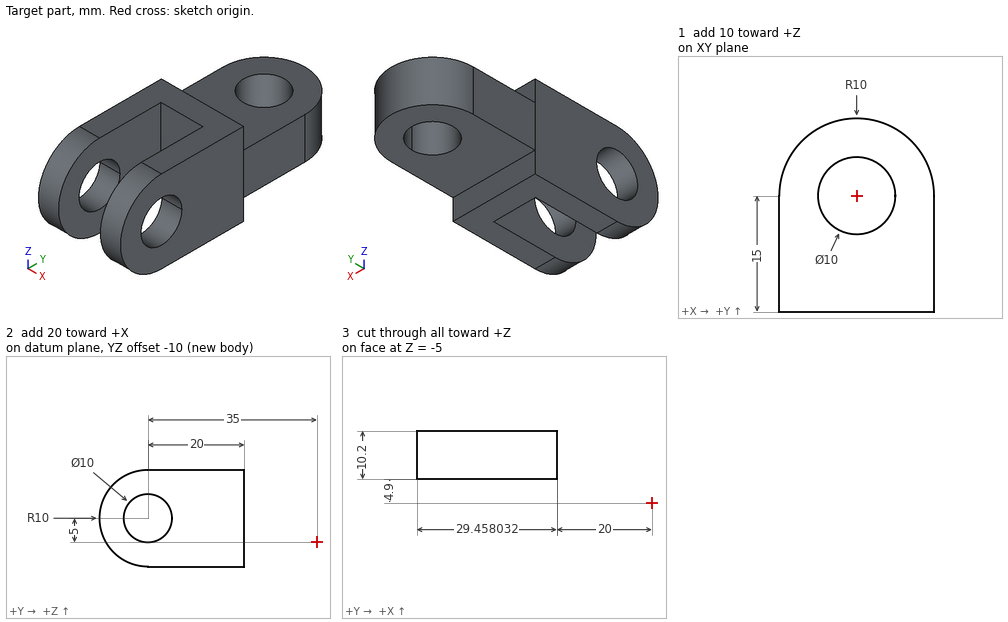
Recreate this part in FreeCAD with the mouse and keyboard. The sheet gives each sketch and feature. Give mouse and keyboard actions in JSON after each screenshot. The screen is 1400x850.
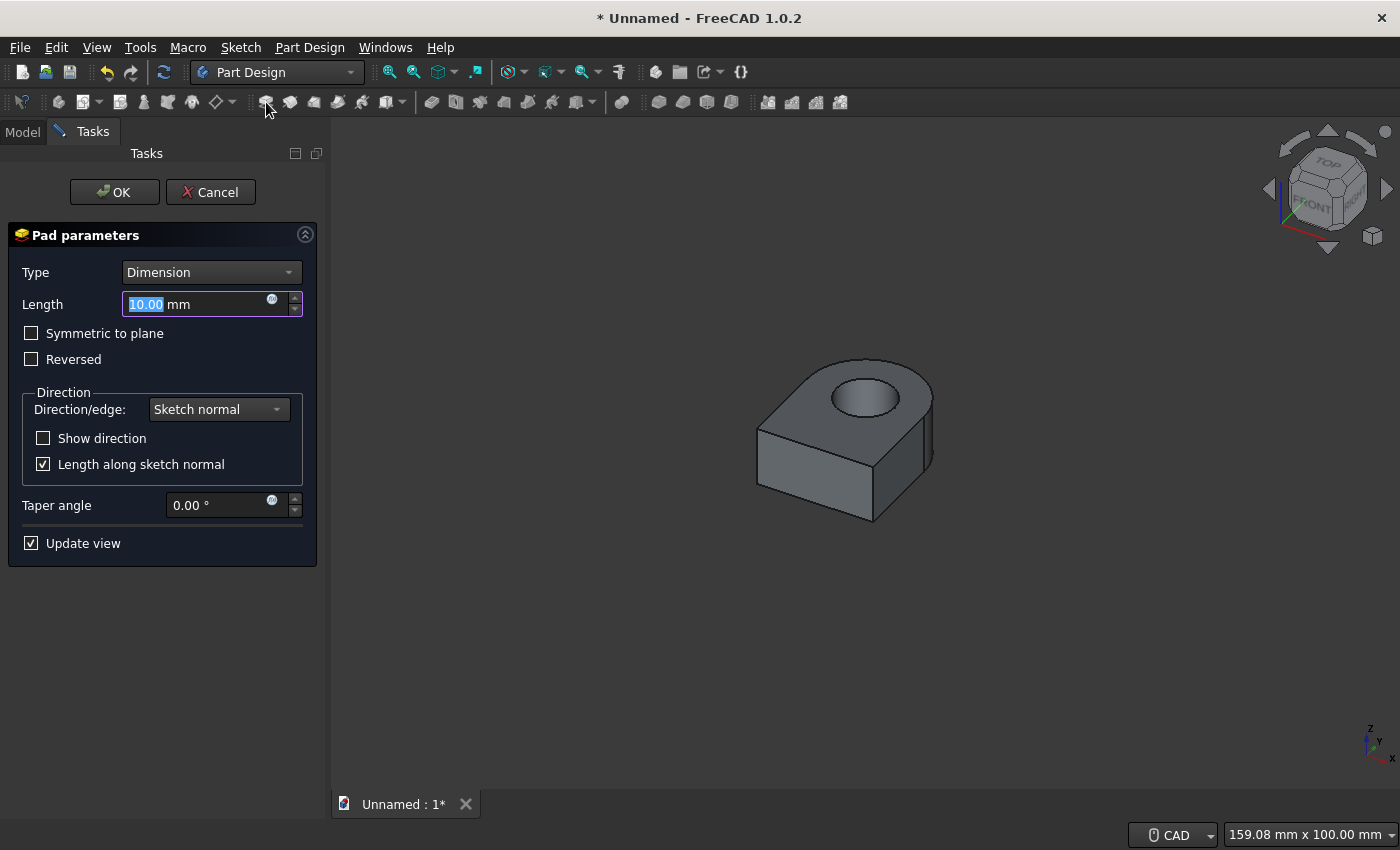
{"action": "type", "text": "10"}
{"action": "key", "text": "Tab"}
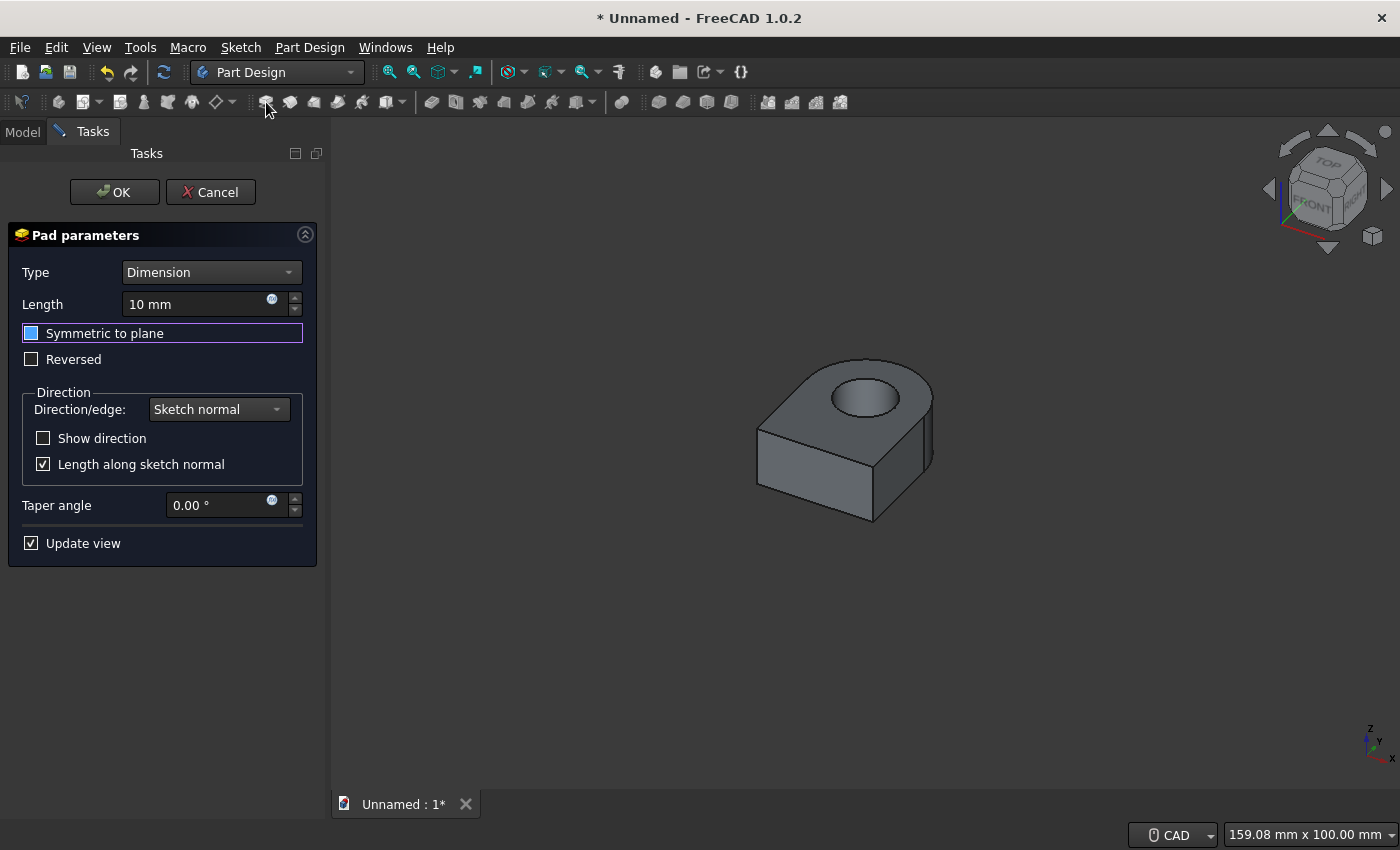
{"action": "left_click", "coordinate": [115, 192]}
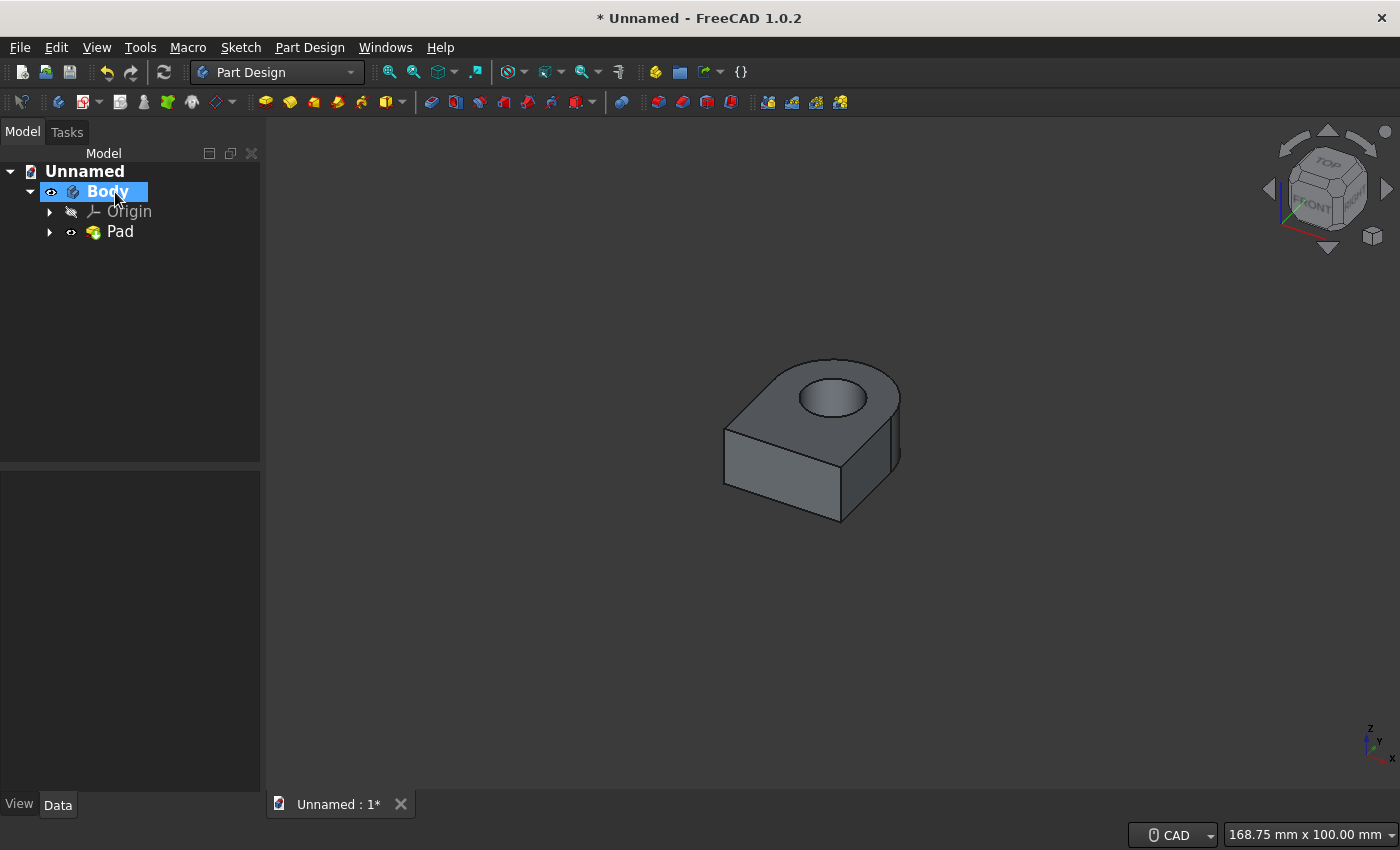
{"action": "left_click", "coordinate": [390, 72]}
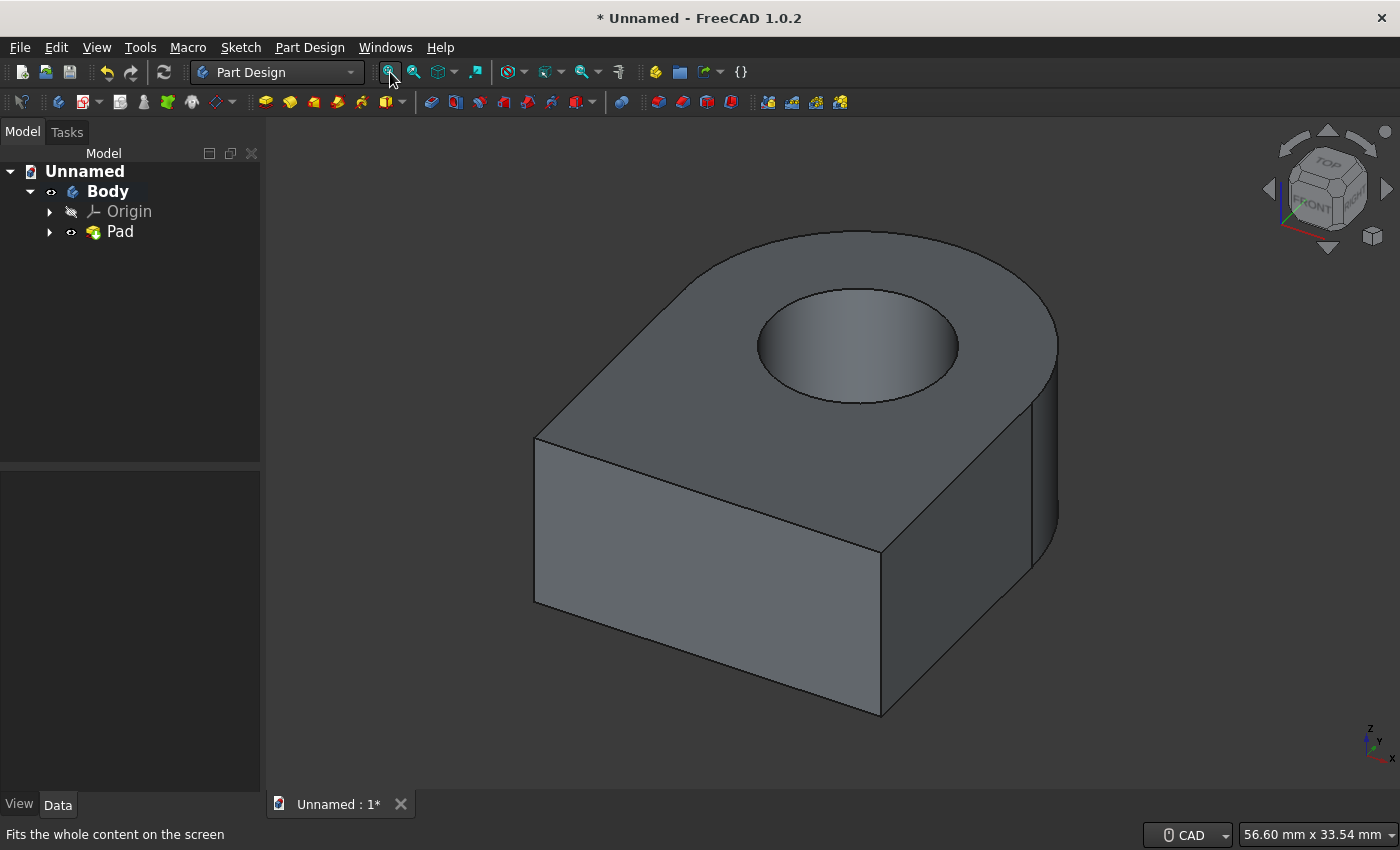
{"action": "left_click", "coordinate": [60, 102]}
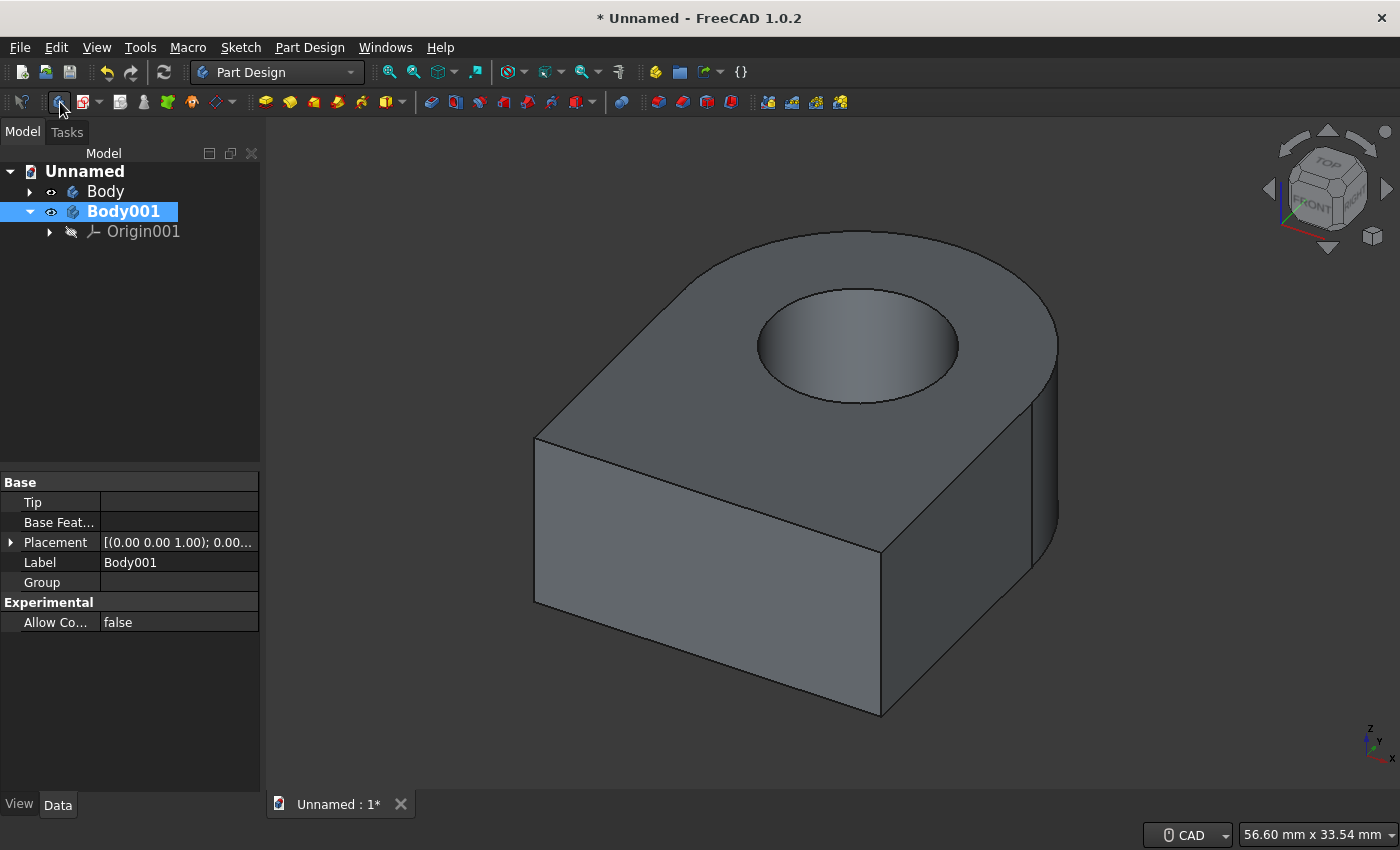
{"action": "left_click", "coordinate": [50, 232]}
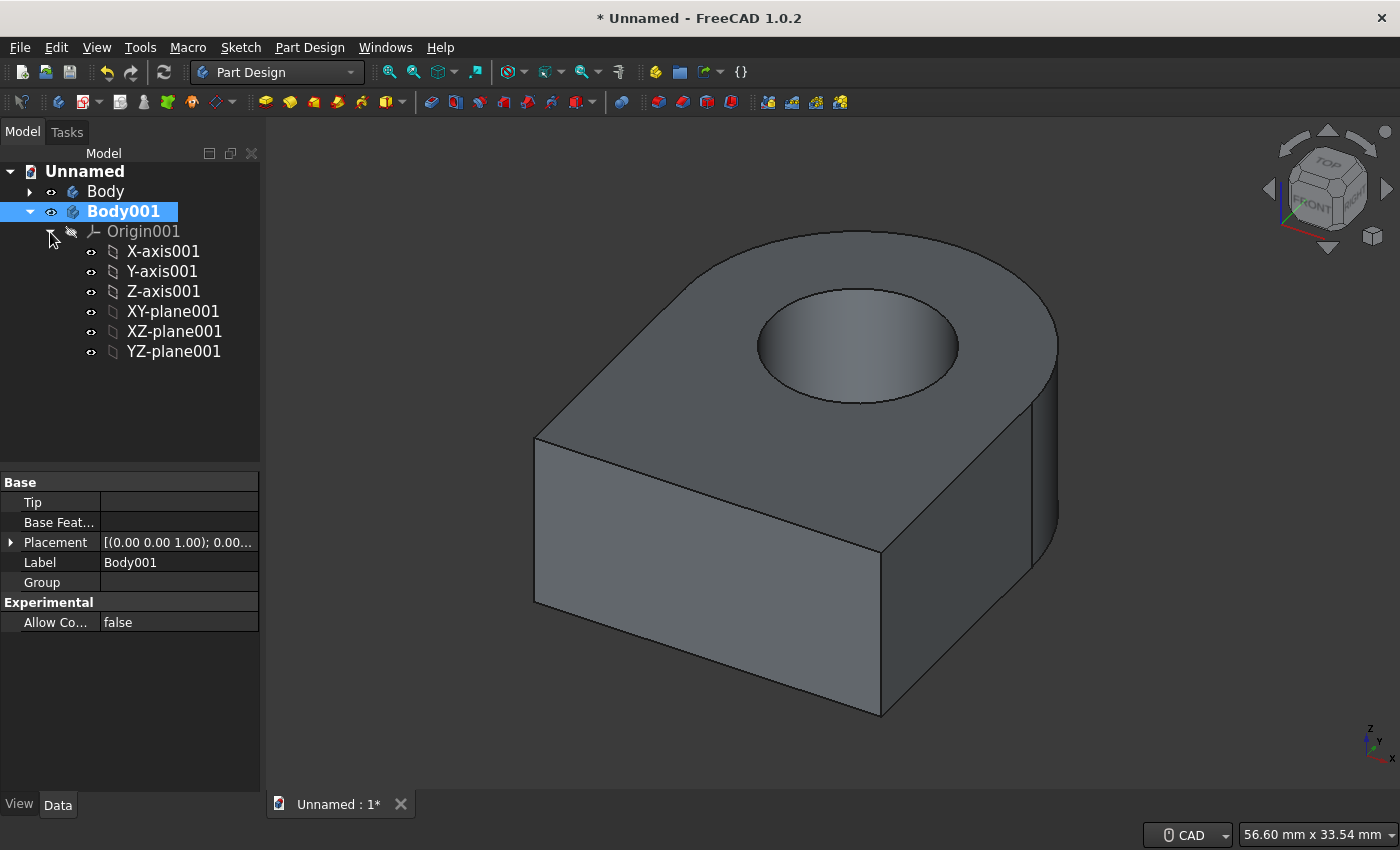
{"action": "left_click", "coordinate": [136, 352]}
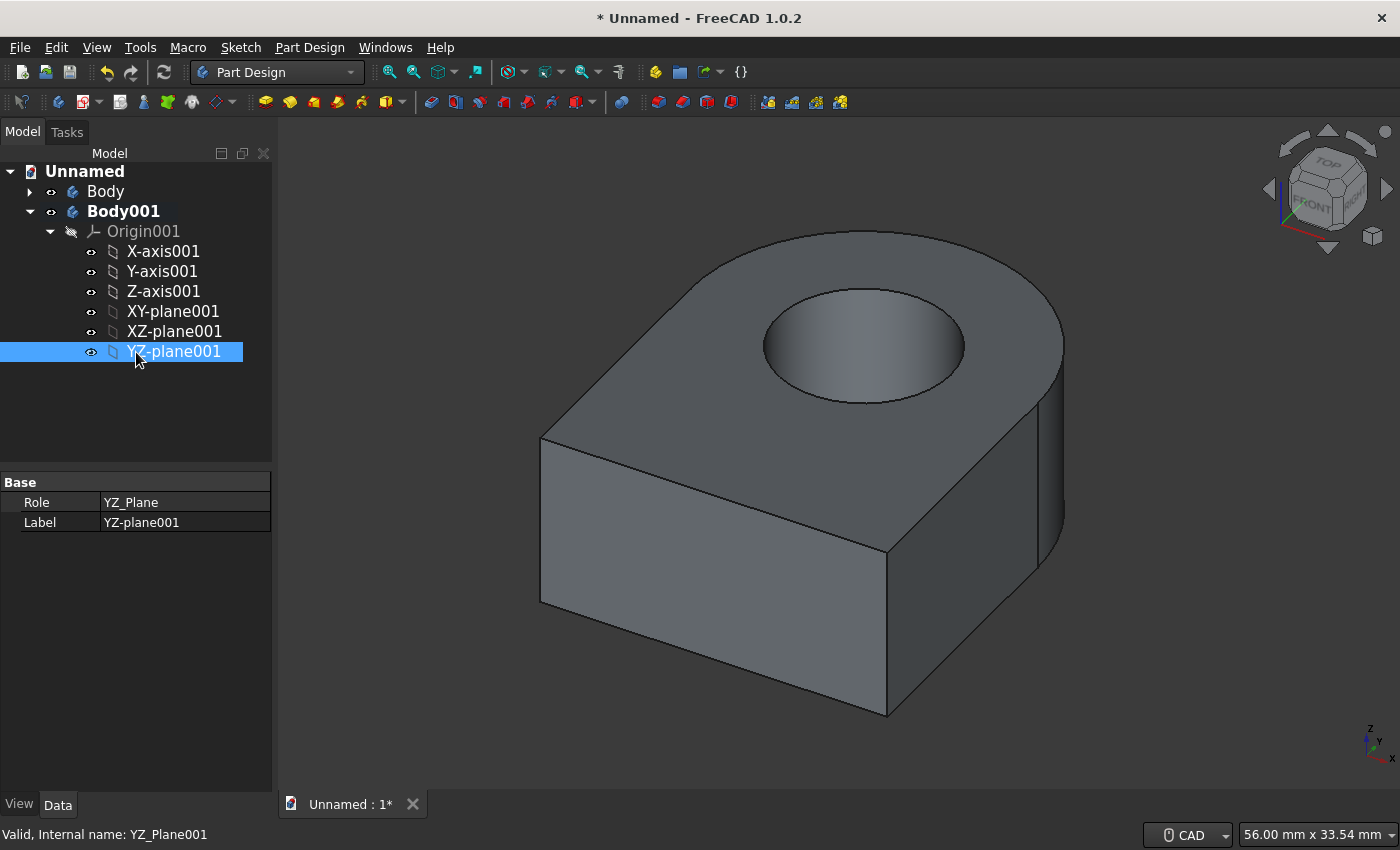
{"action": "left_click", "coordinate": [216, 102]}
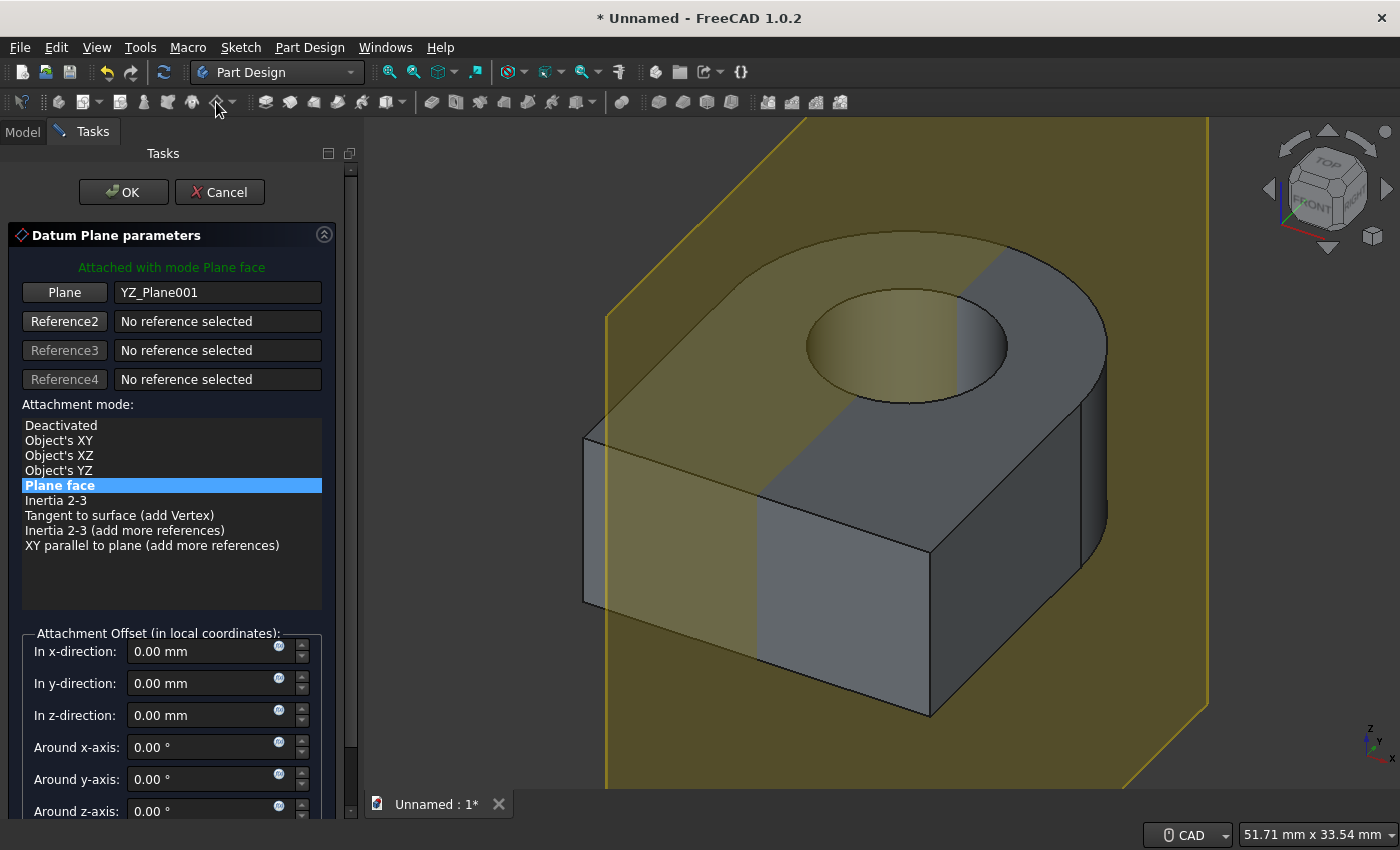
{"action": "triple_click", "coordinate": [210, 715]}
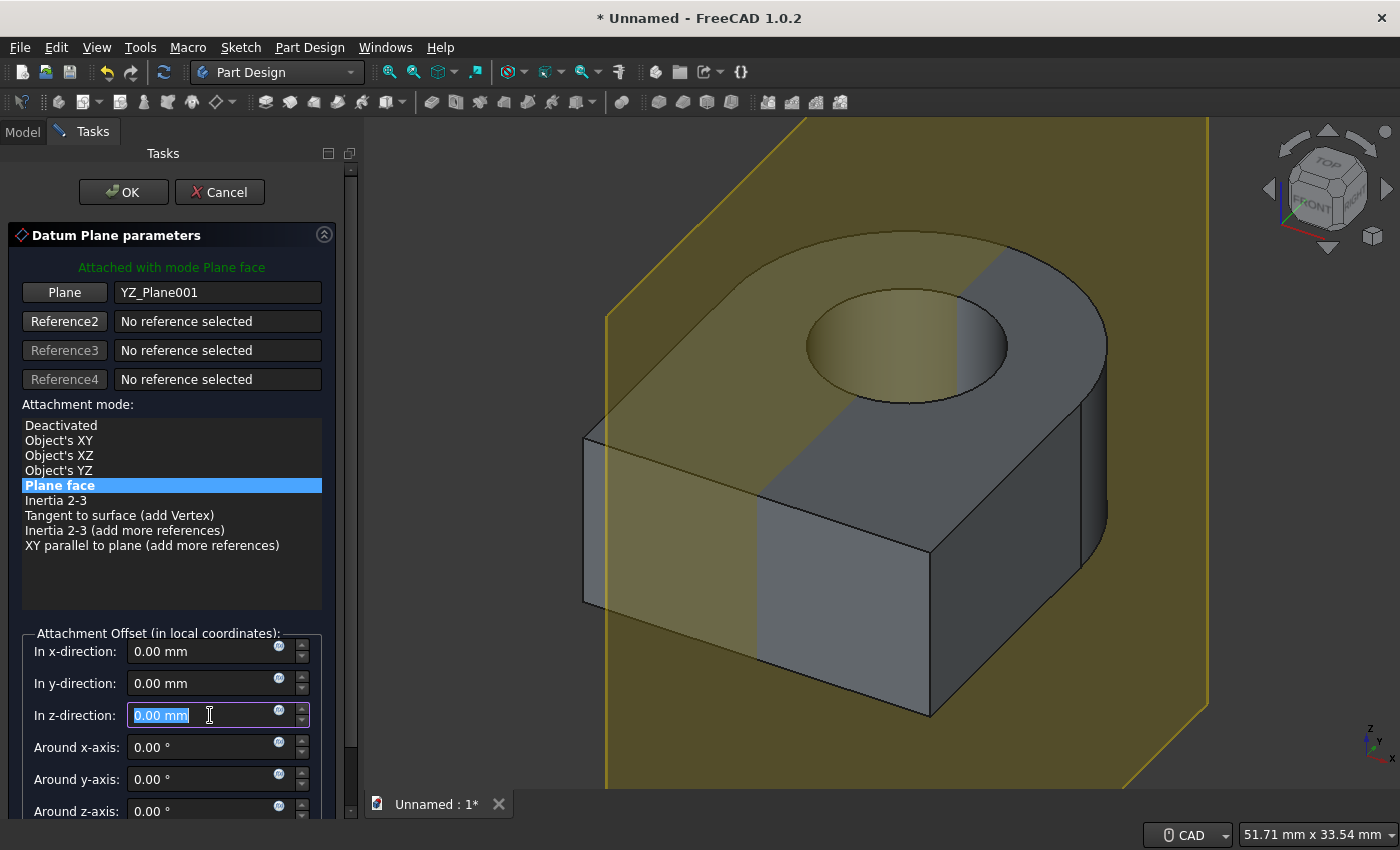
{"action": "type", "text": "-10"}
{"action": "key", "text": "Tab"}